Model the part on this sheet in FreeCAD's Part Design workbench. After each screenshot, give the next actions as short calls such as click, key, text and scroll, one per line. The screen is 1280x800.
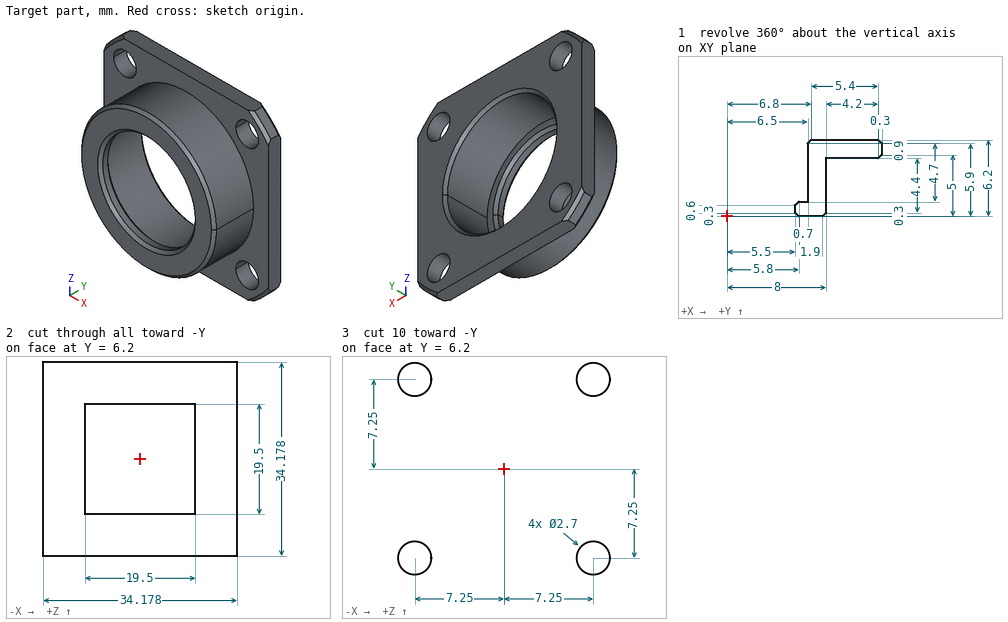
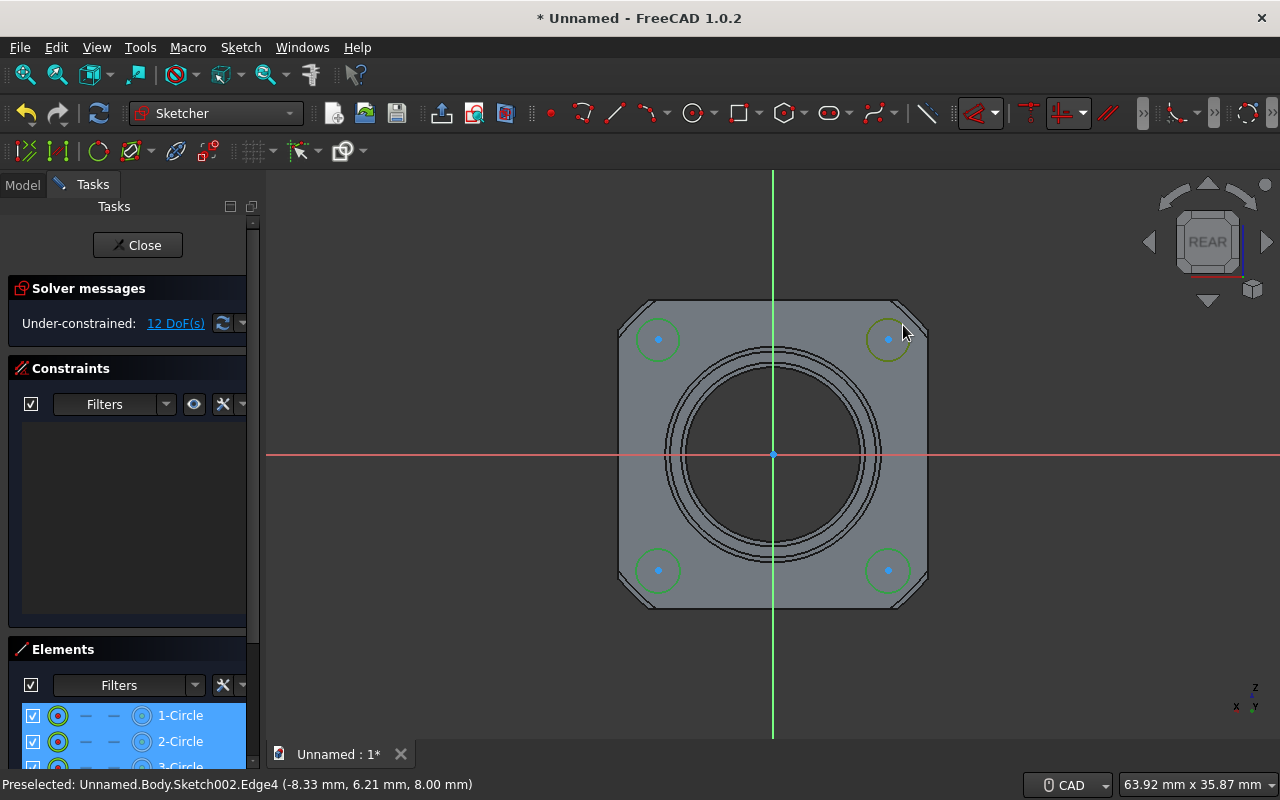
key(e)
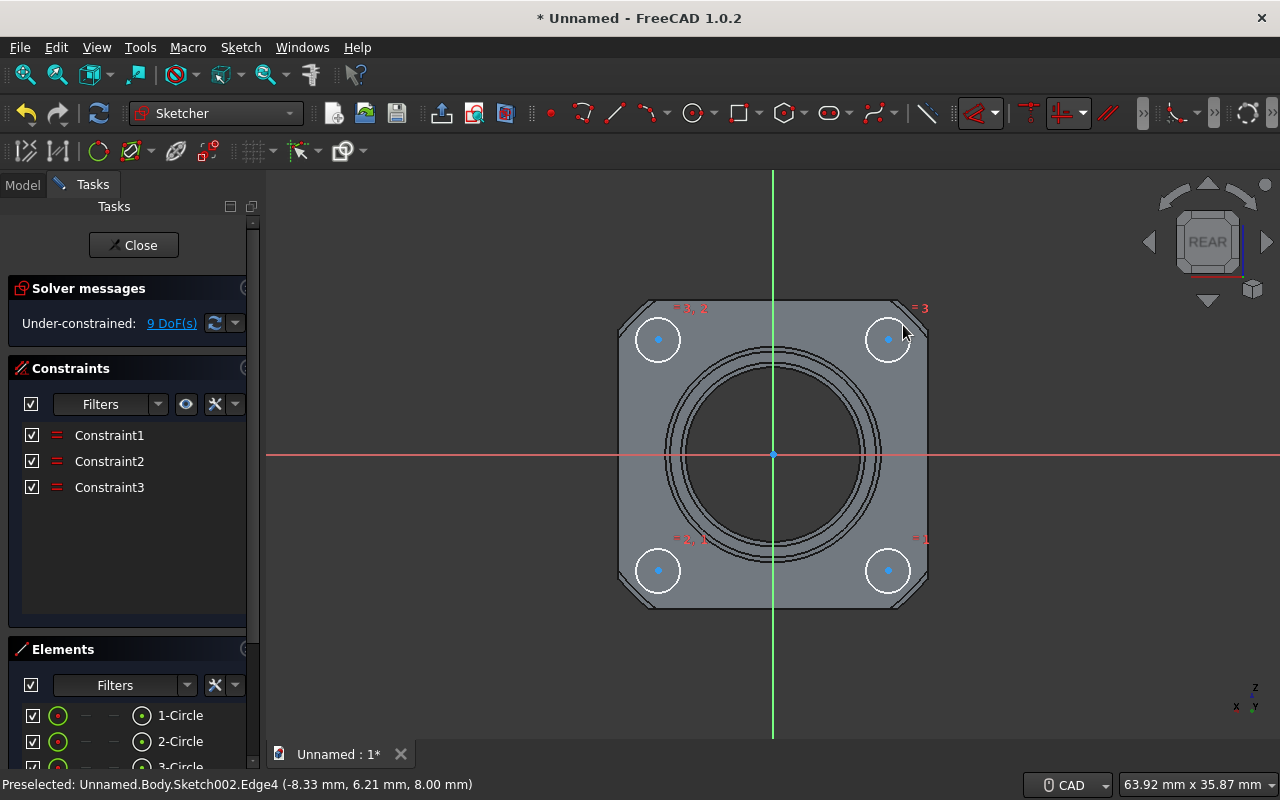
click(888, 571)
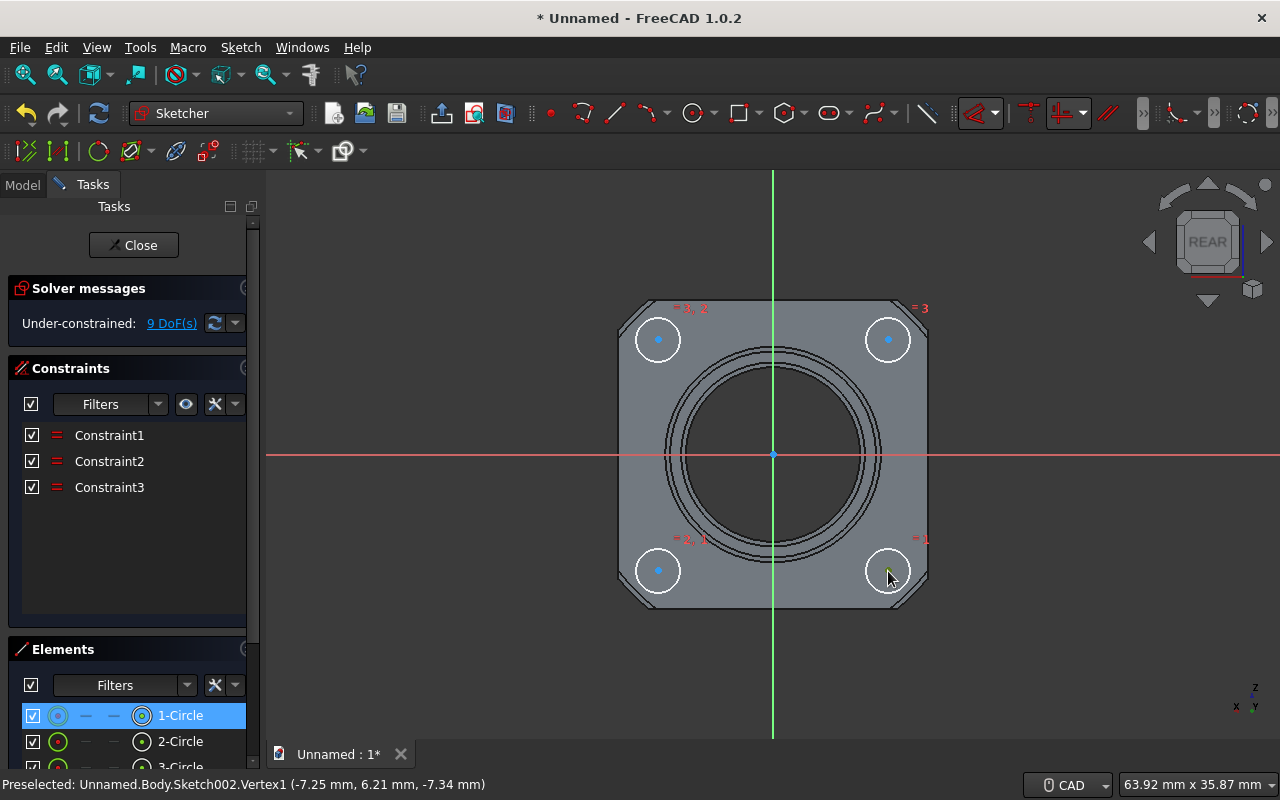
click(658, 571)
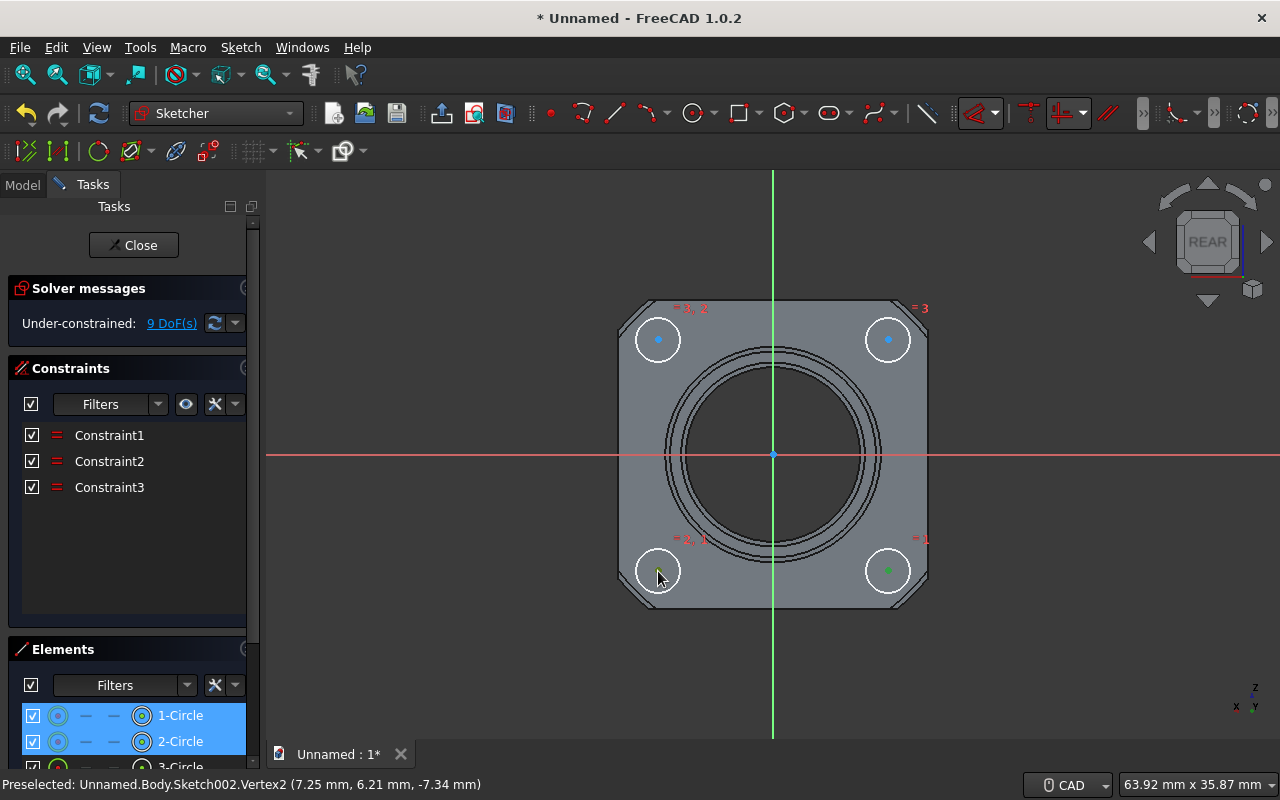
click(1086, 114)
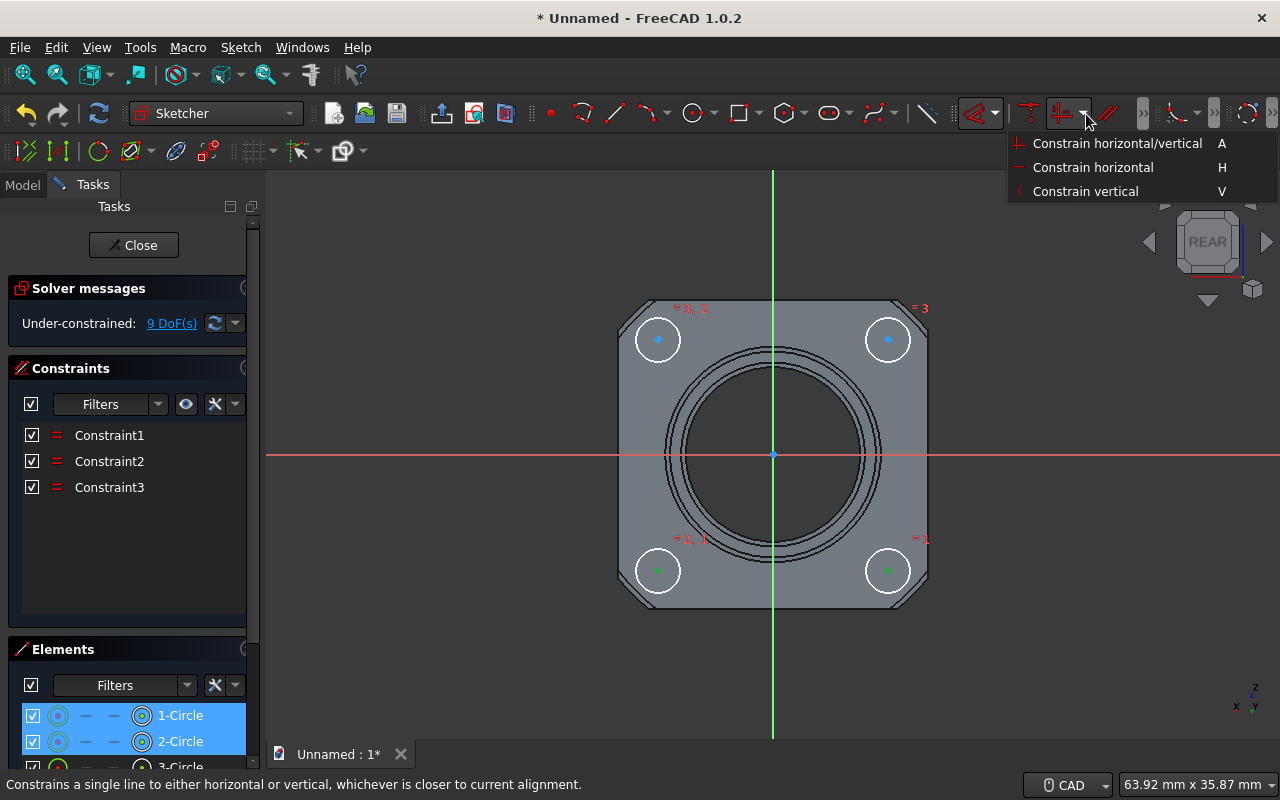
click(1143, 167)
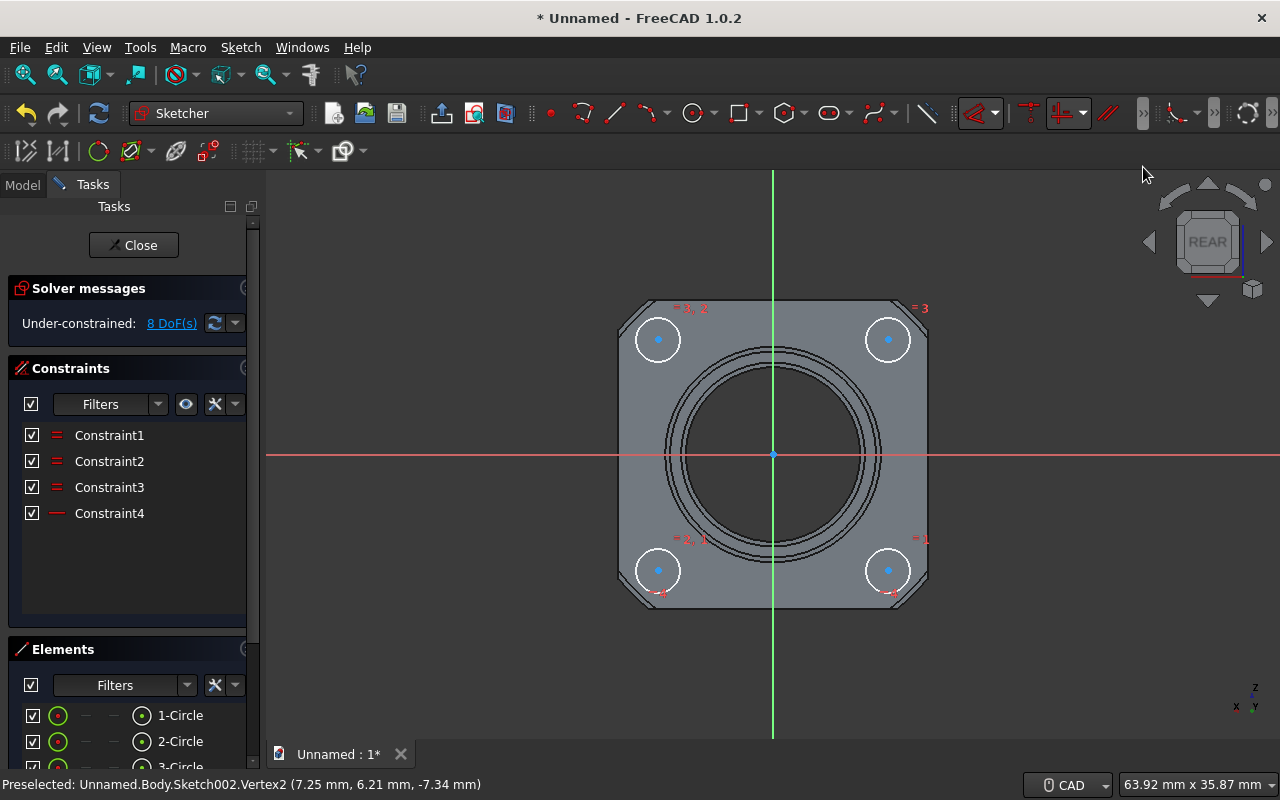
click(658, 571)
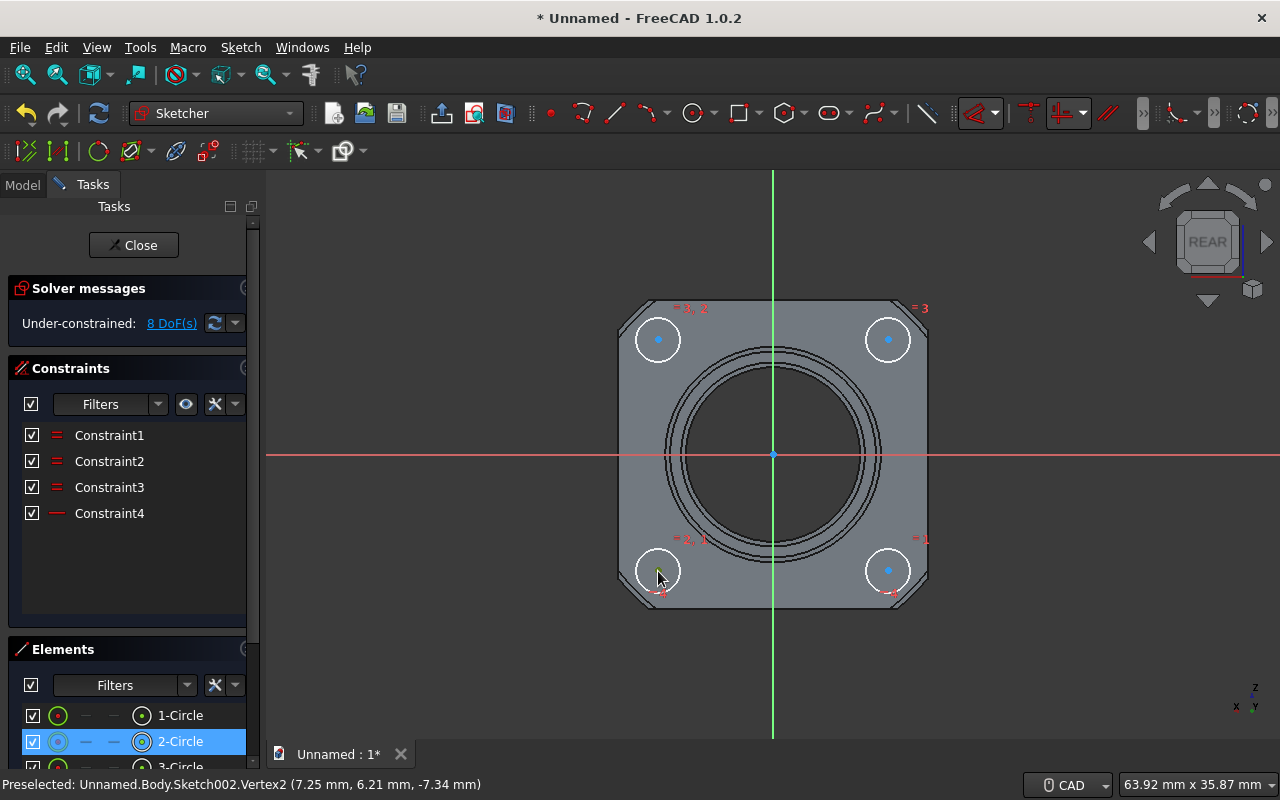
click(658, 340)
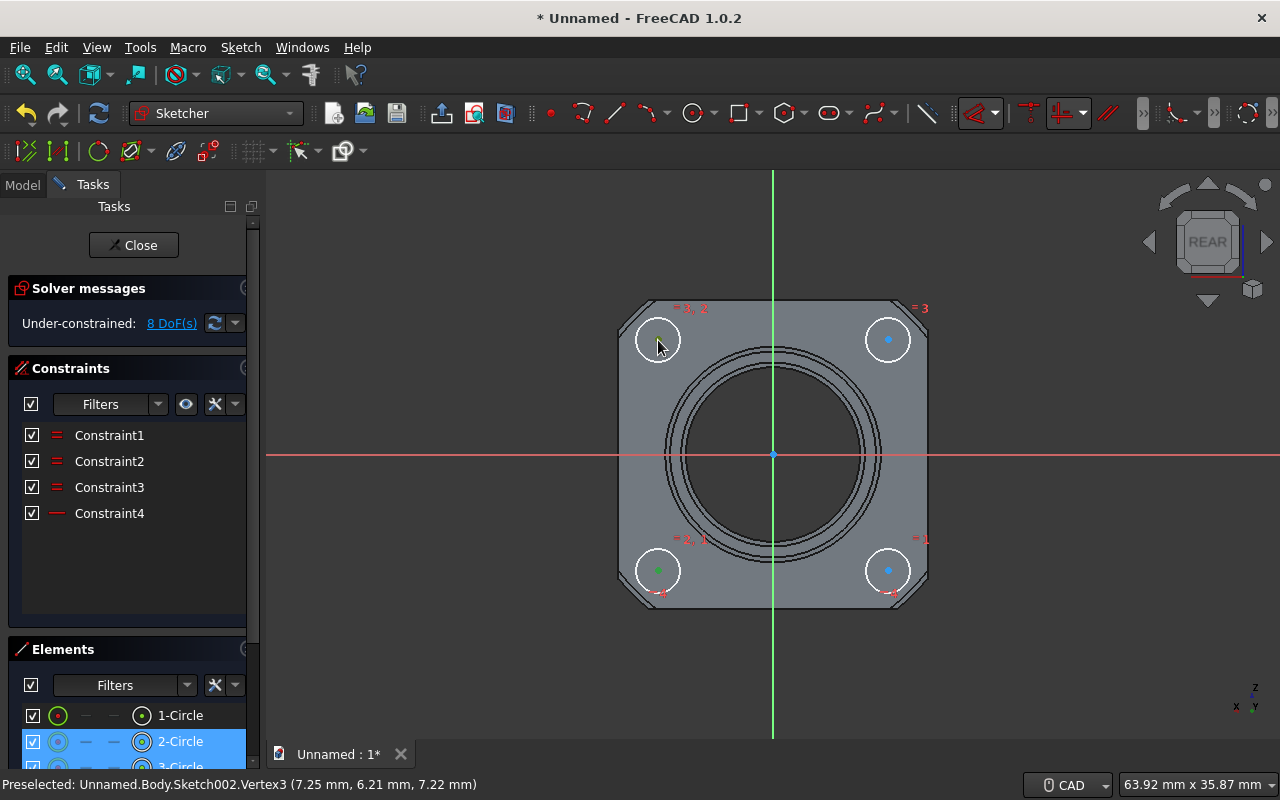
click(1086, 114)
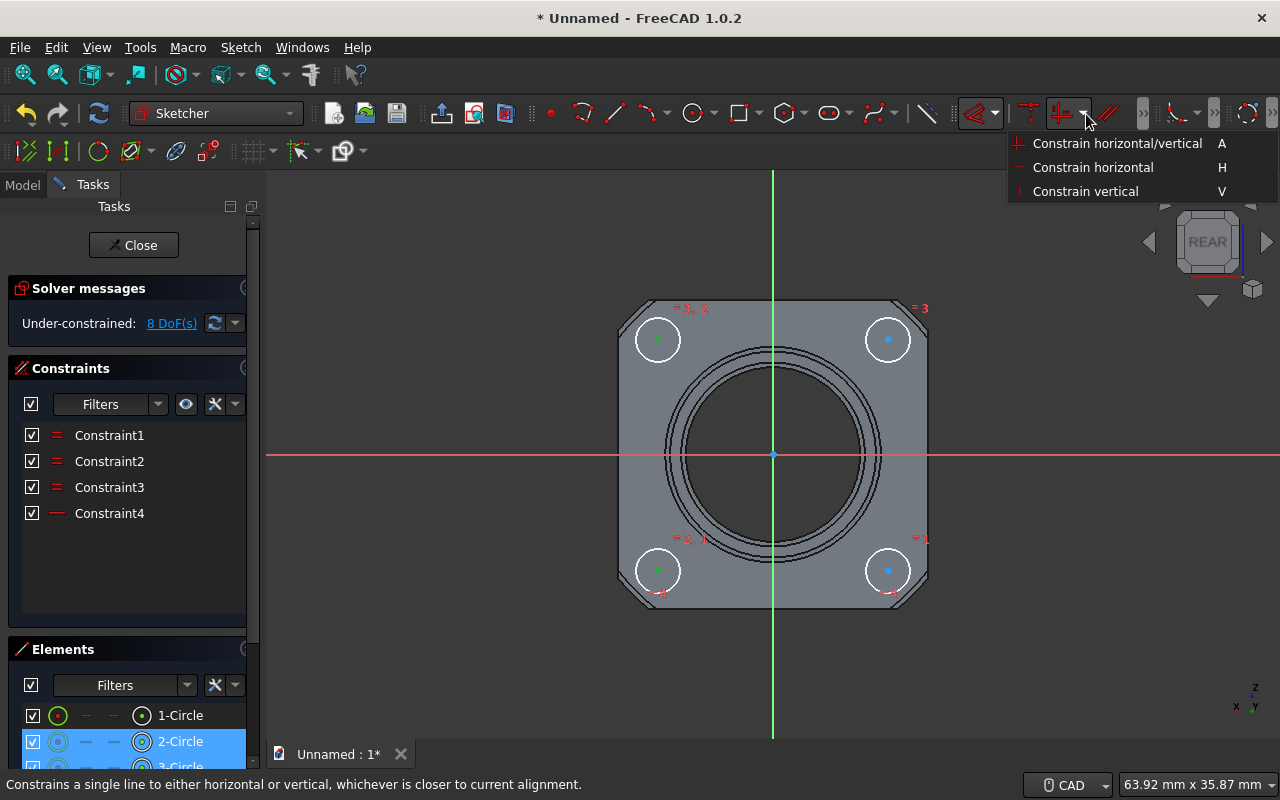
click(1143, 191)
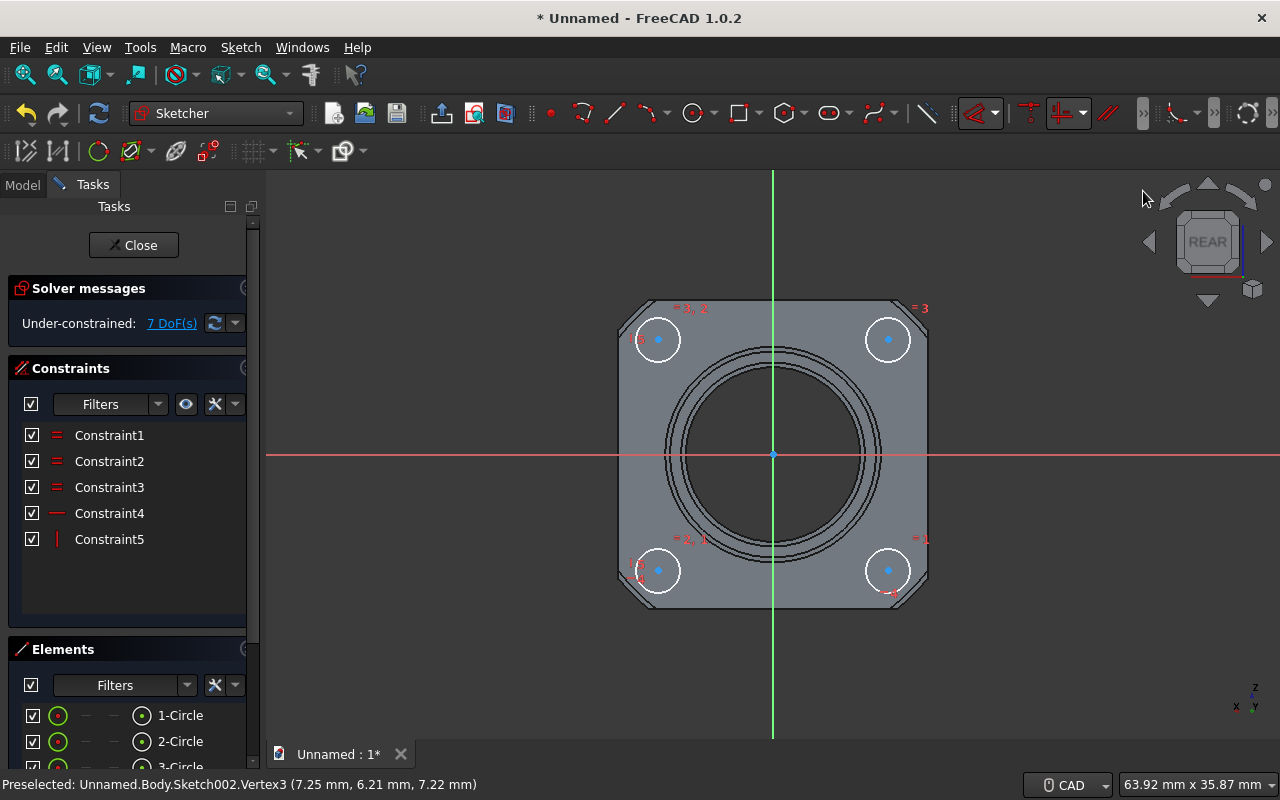
click(888, 571)